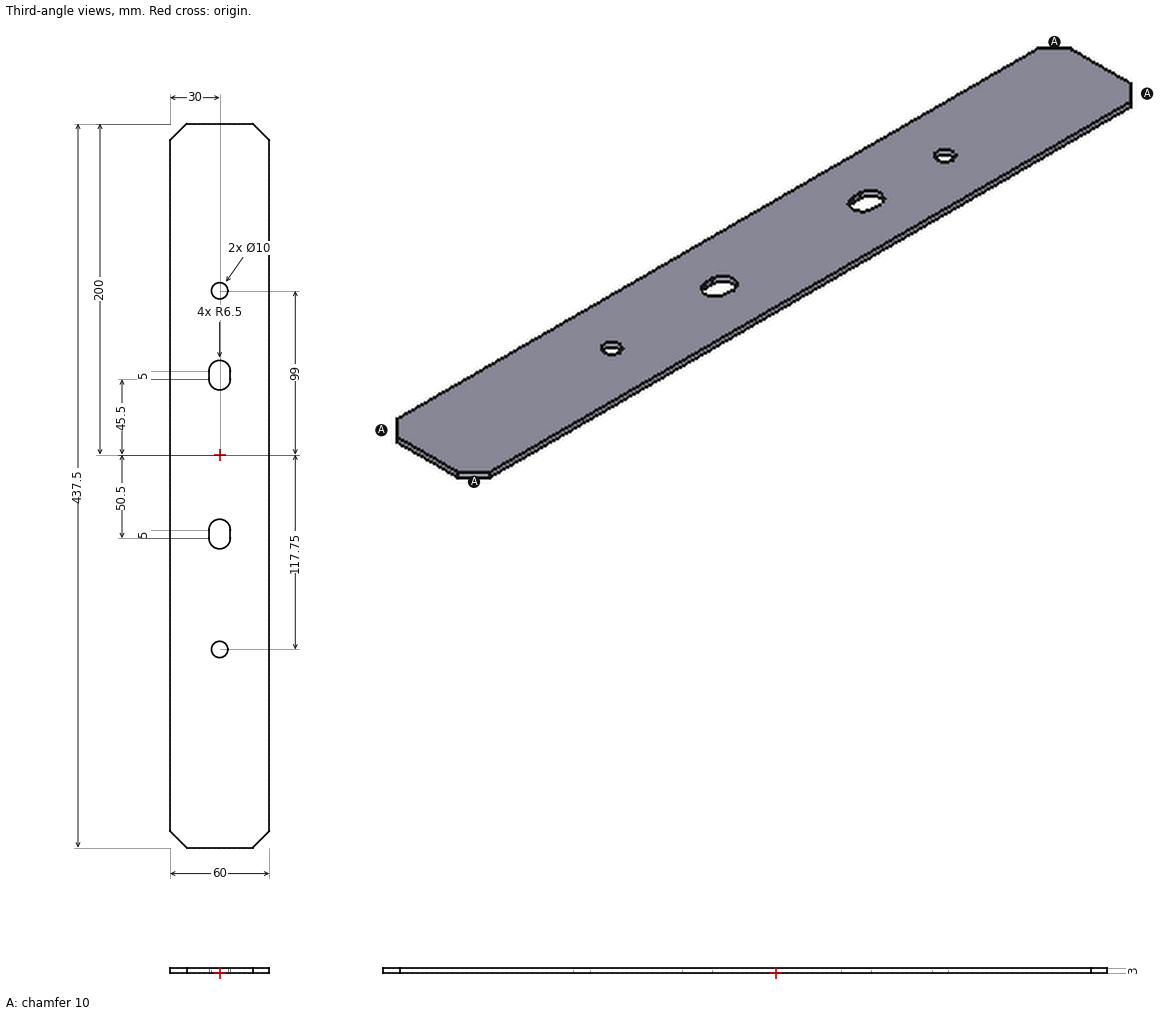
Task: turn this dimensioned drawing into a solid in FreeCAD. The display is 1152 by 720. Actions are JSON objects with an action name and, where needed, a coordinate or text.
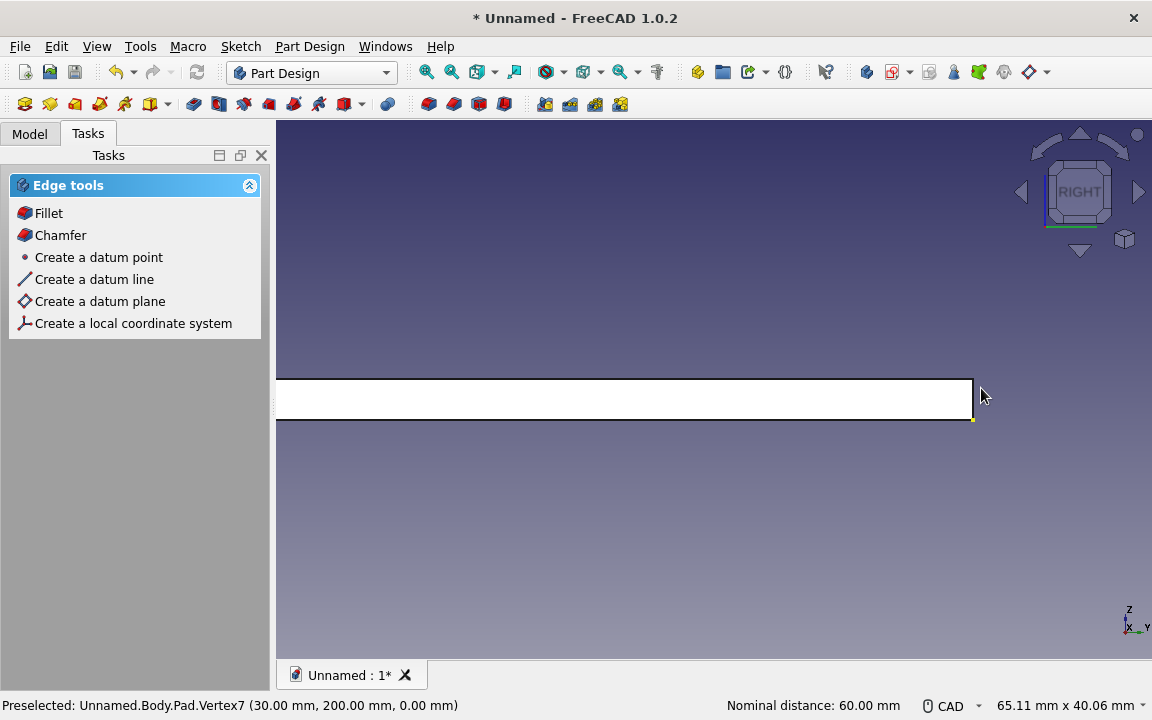
{"action": "left_click", "coordinate": [973, 399], "text": "ctrl"}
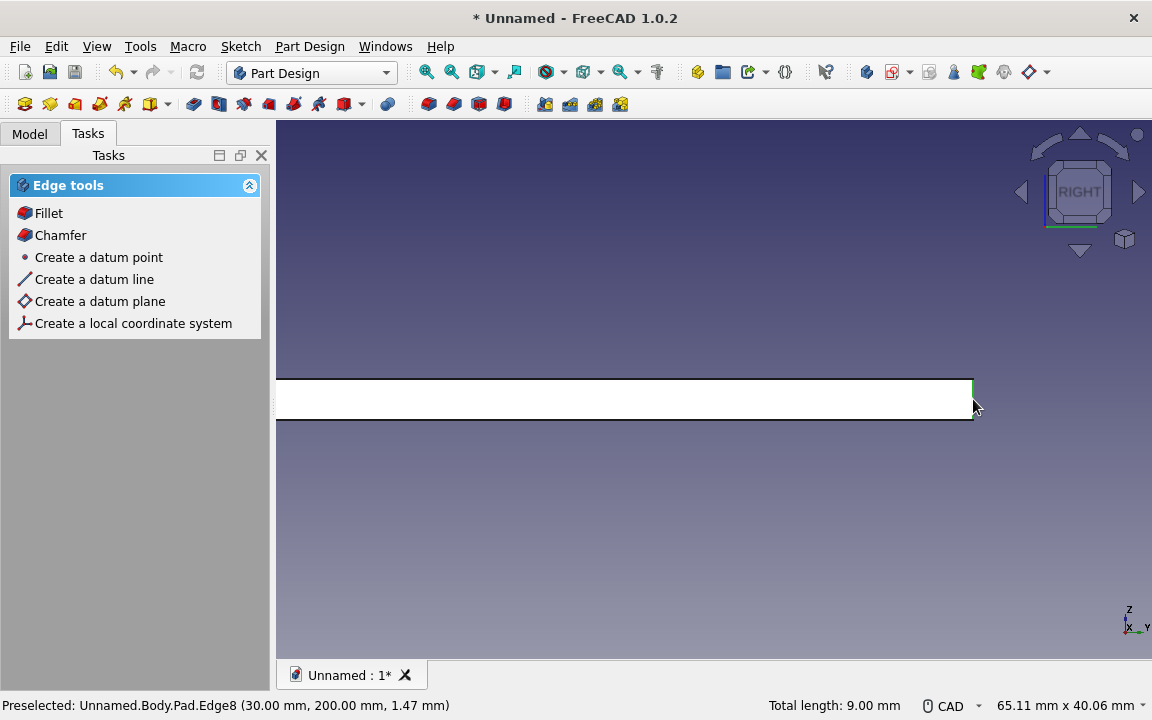
{"action": "left_click", "coordinate": [427, 72]}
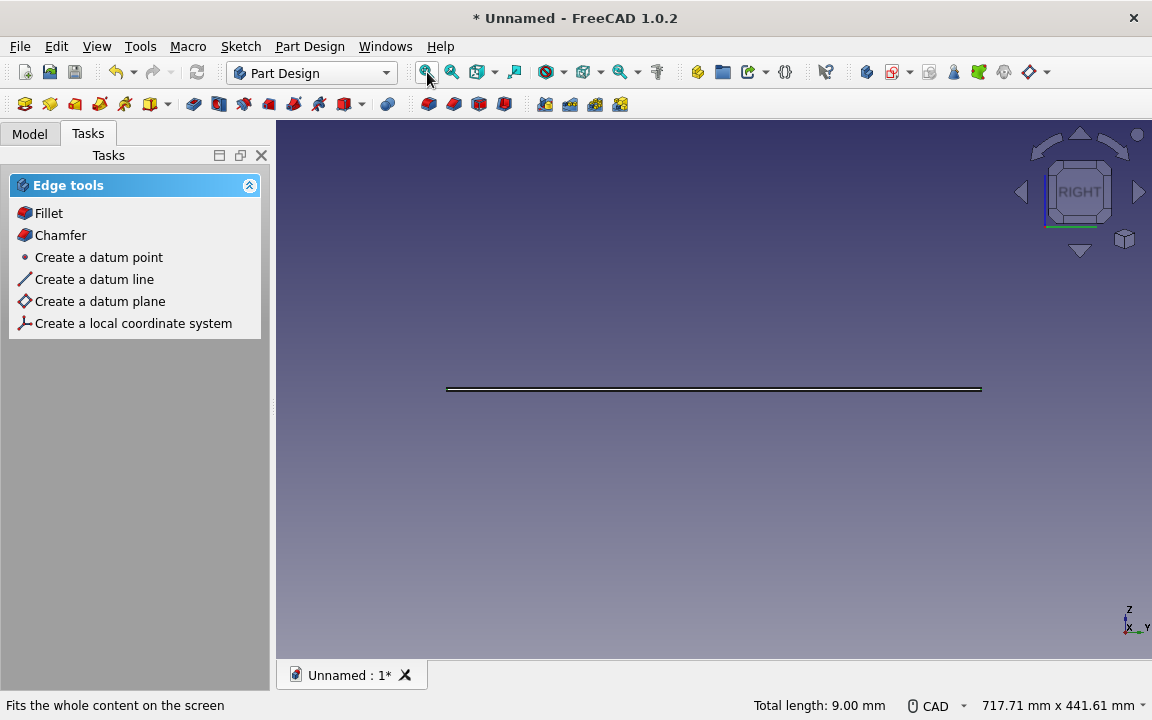
{"action": "key", "text": "5"}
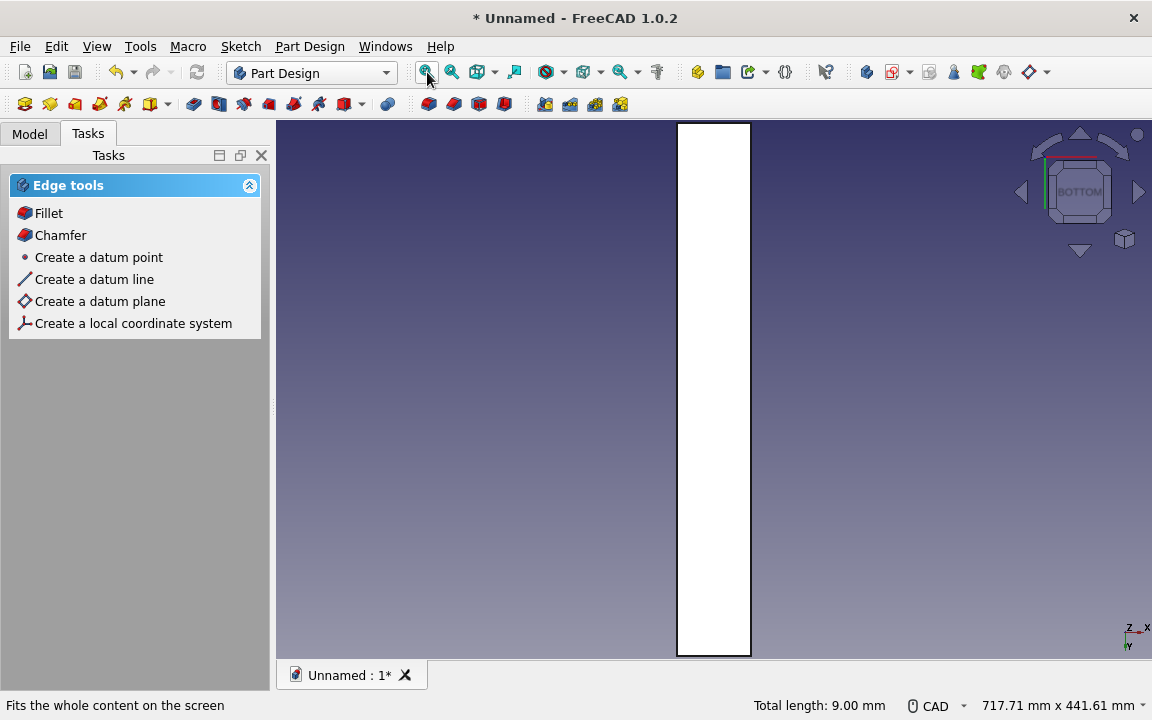
{"action": "key", "text": "4"}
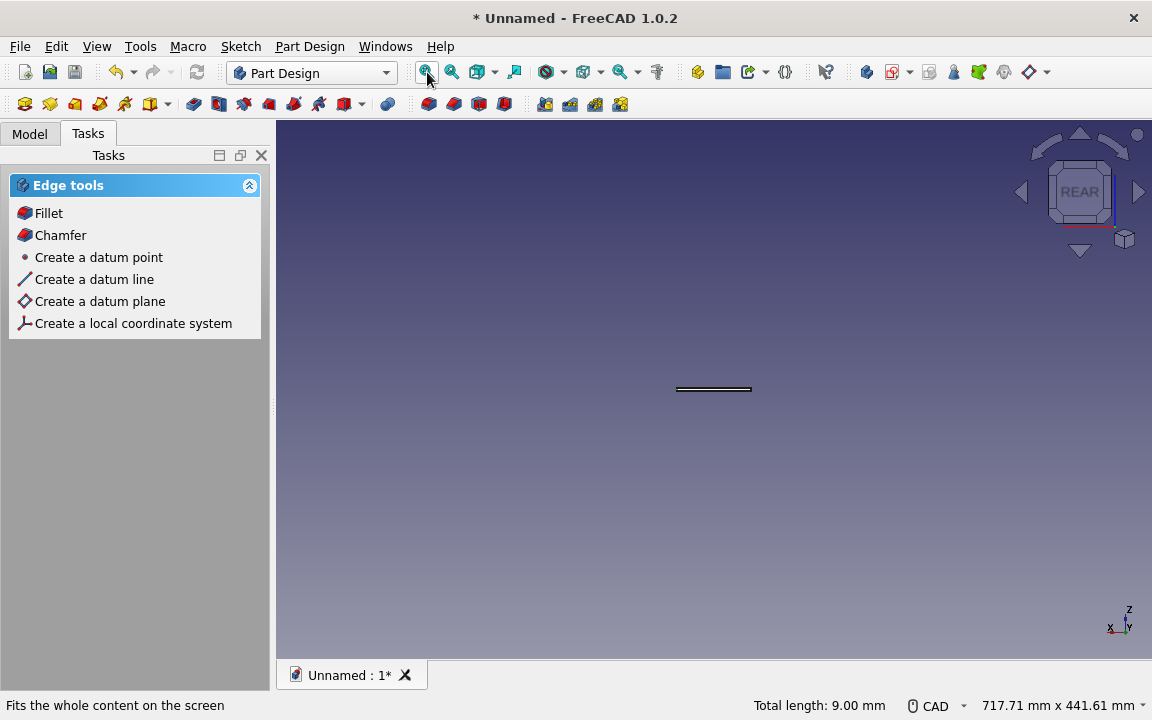
{"action": "left_click", "coordinate": [427, 72]}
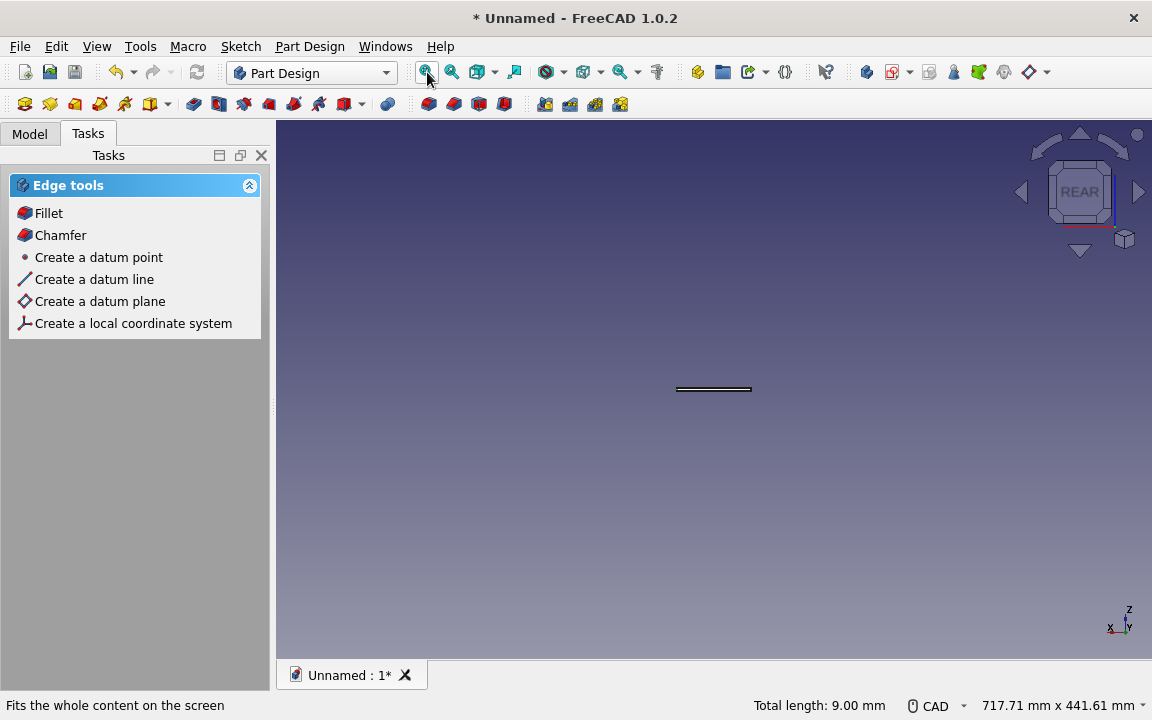
{"action": "scroll", "coordinate": [751, 389], "scroll_direction": "up", "scroll_amount": 12}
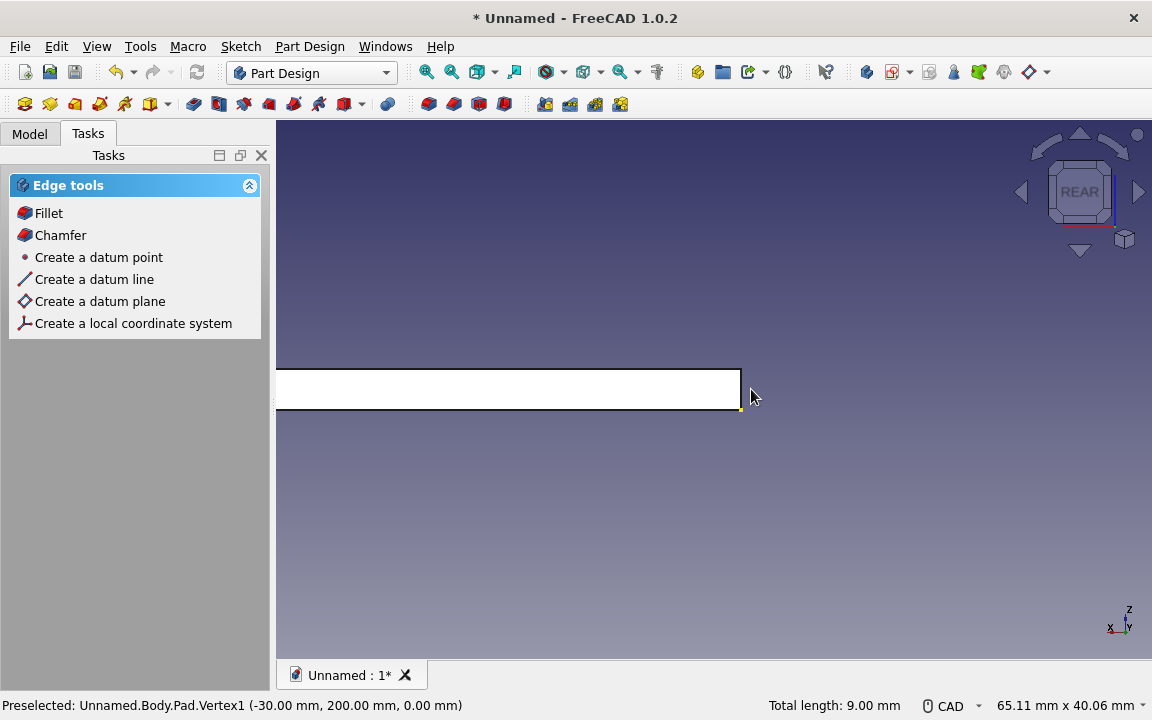
{"action": "left_click", "coordinate": [741, 389], "text": "ctrl"}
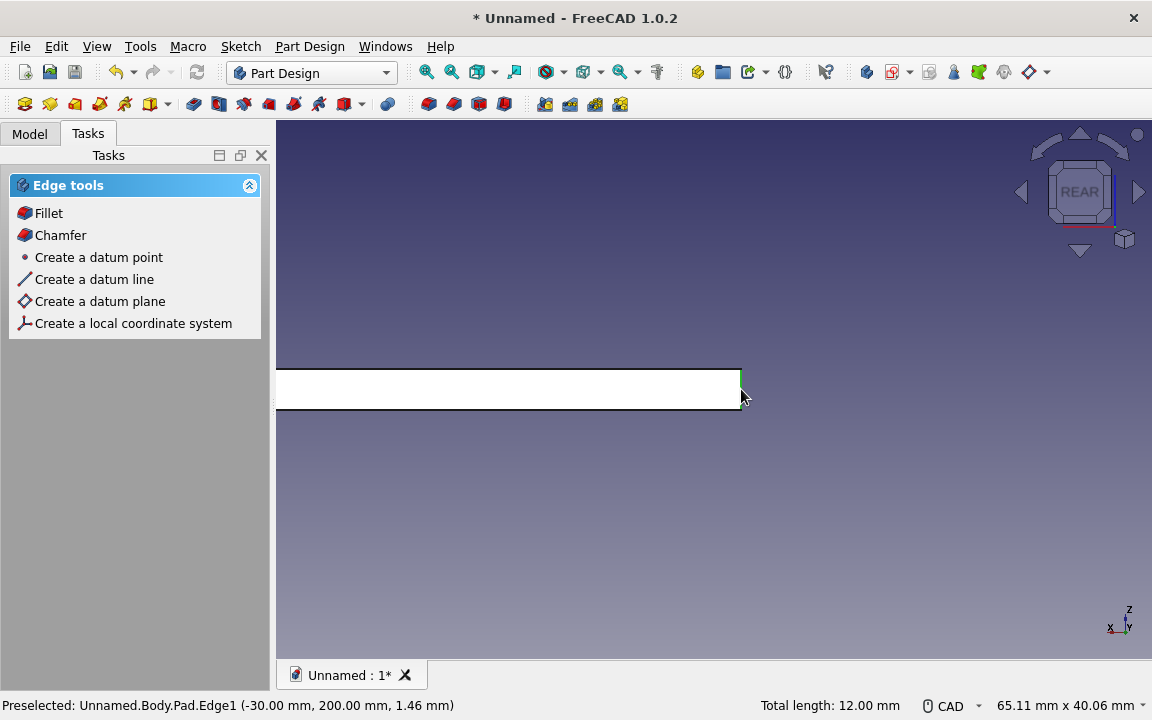
{"action": "left_click", "coordinate": [454, 104]}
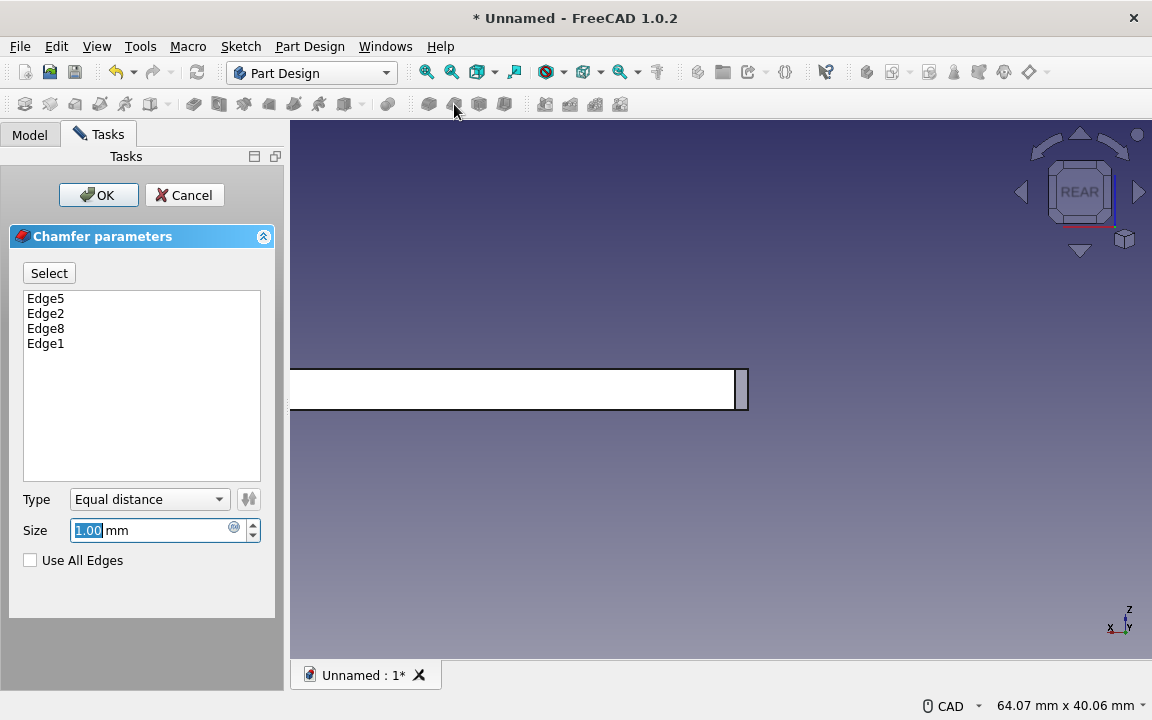
{"action": "type", "text": "10"}
{"action": "key", "text": "Tab"}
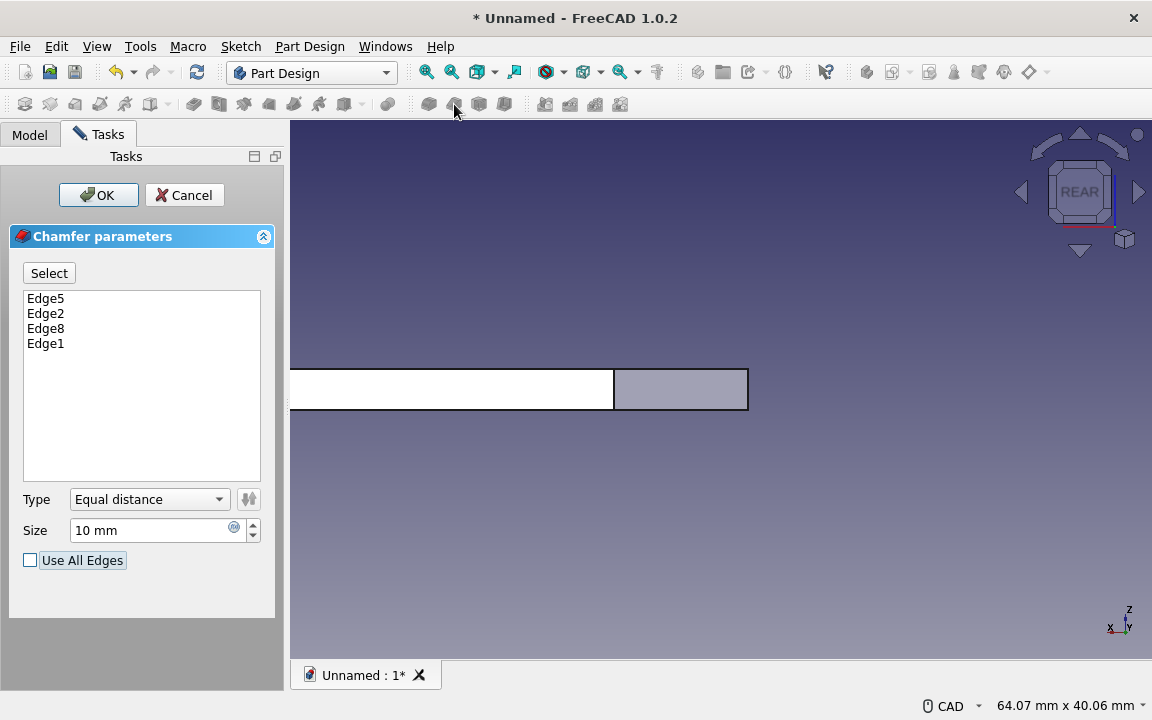
{"action": "left_click", "coordinate": [99, 195]}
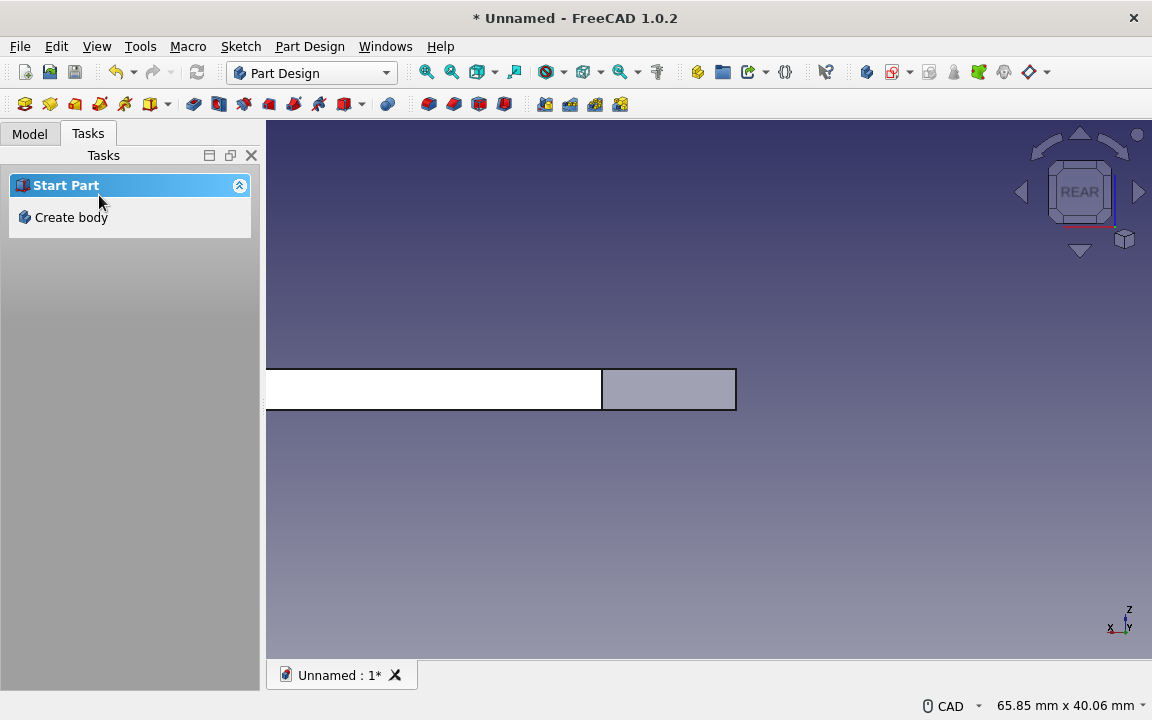
{"action": "left_click", "coordinate": [427, 72]}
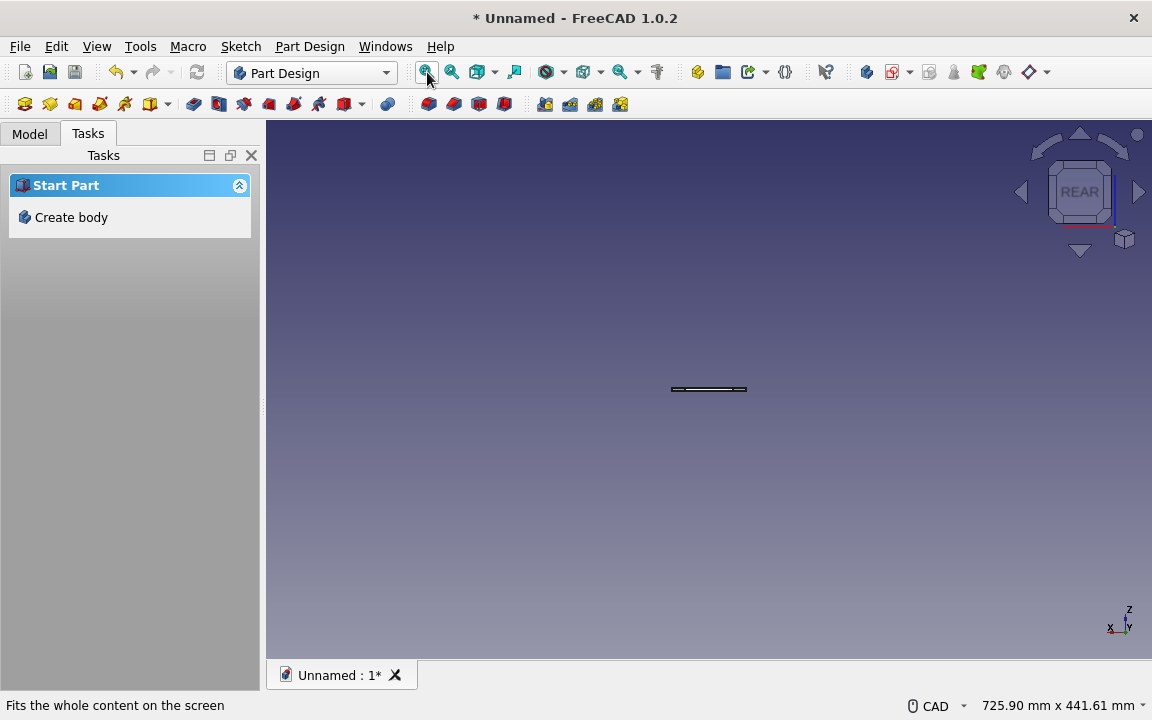
{"action": "key", "text": "0"}